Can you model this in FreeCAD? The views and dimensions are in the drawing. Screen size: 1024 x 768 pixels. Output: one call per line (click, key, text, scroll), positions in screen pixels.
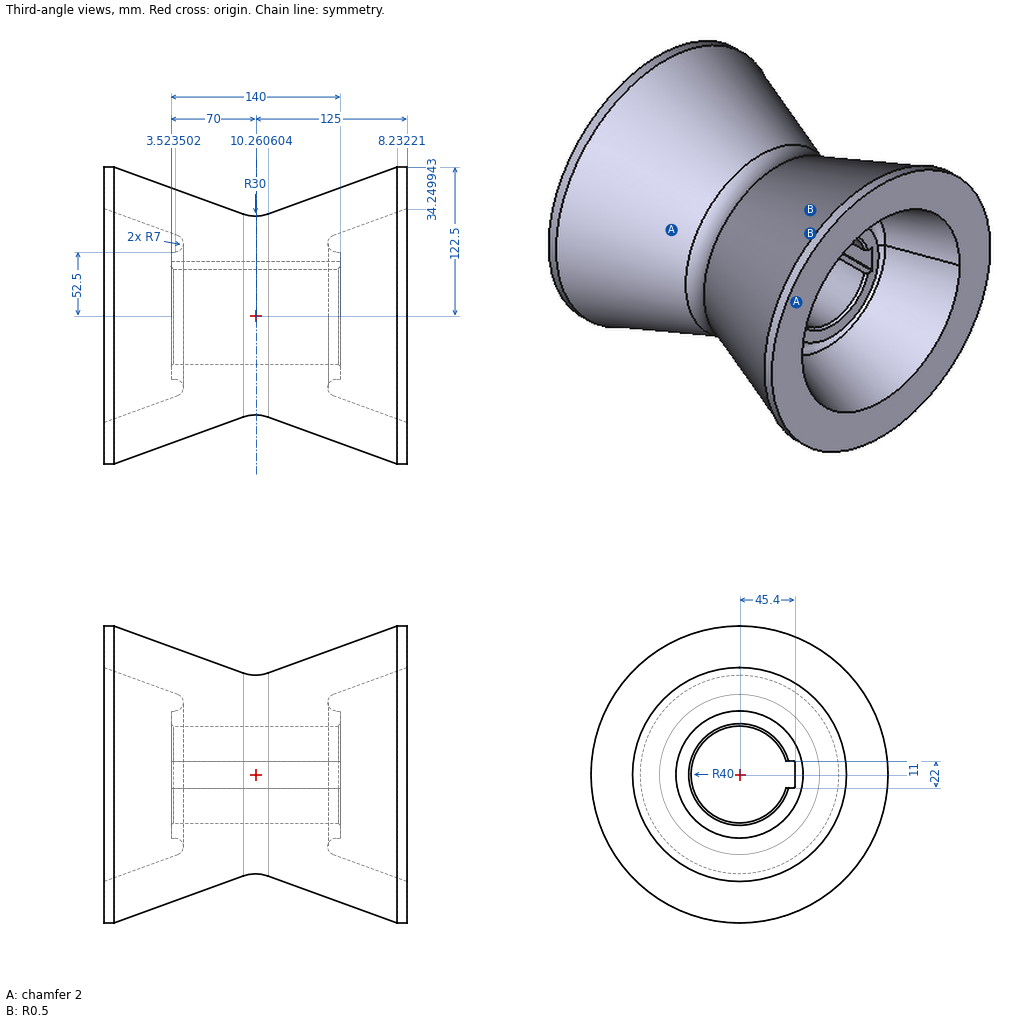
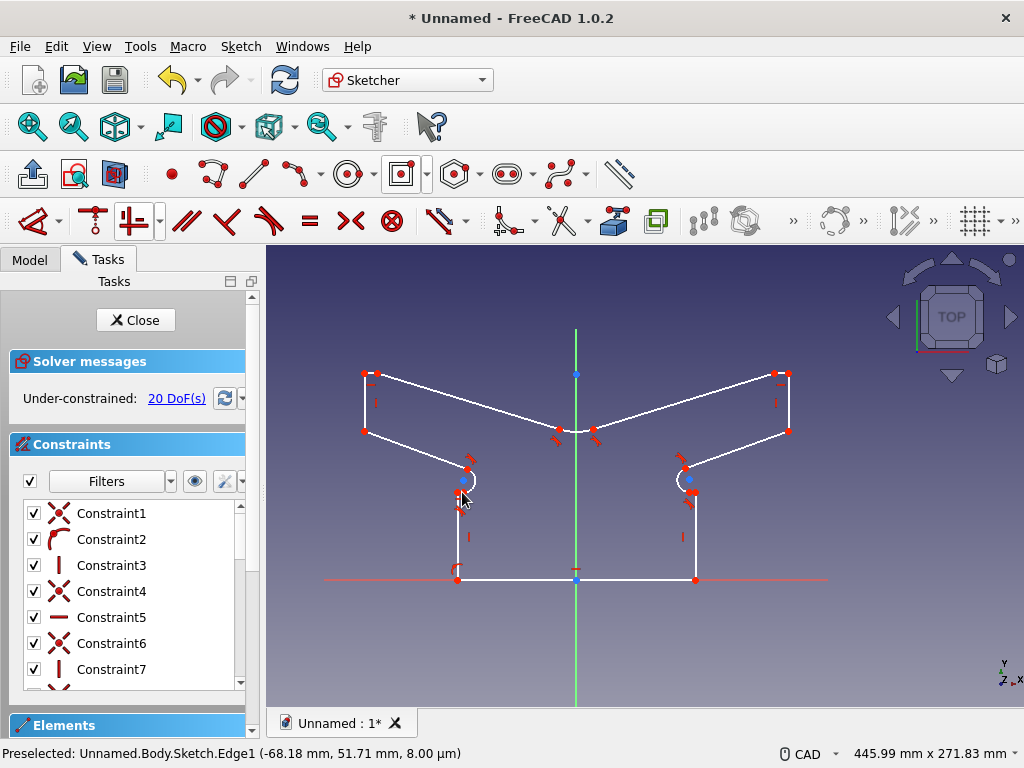
scroll(693, 492, up, 9)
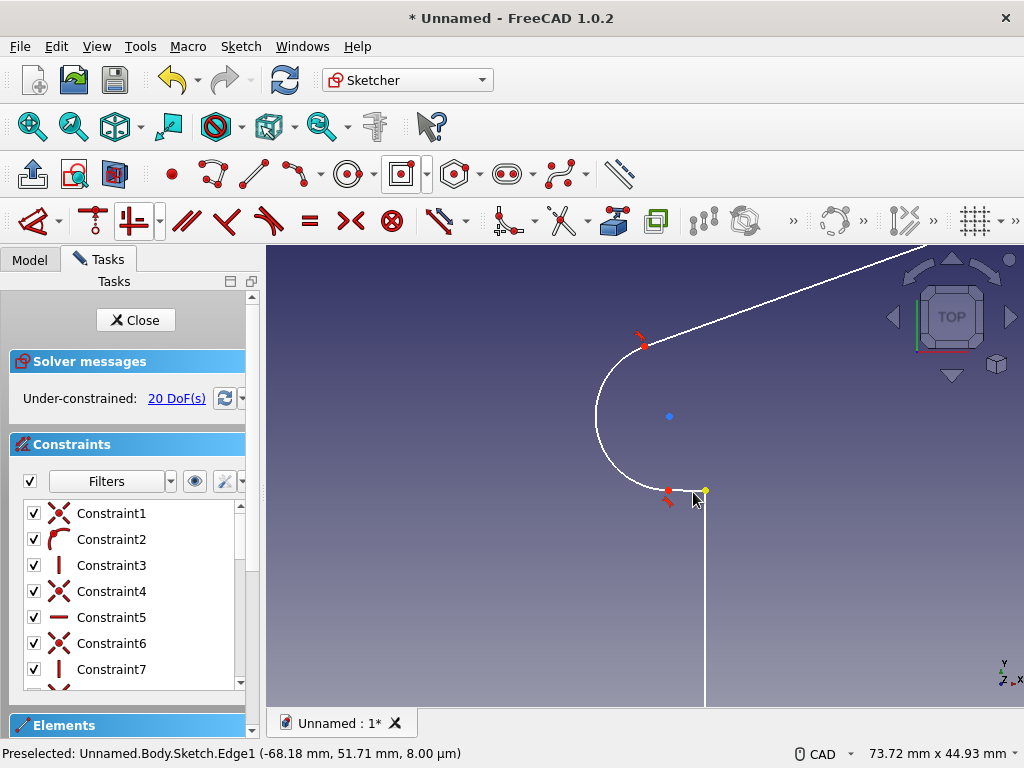
click(691, 491)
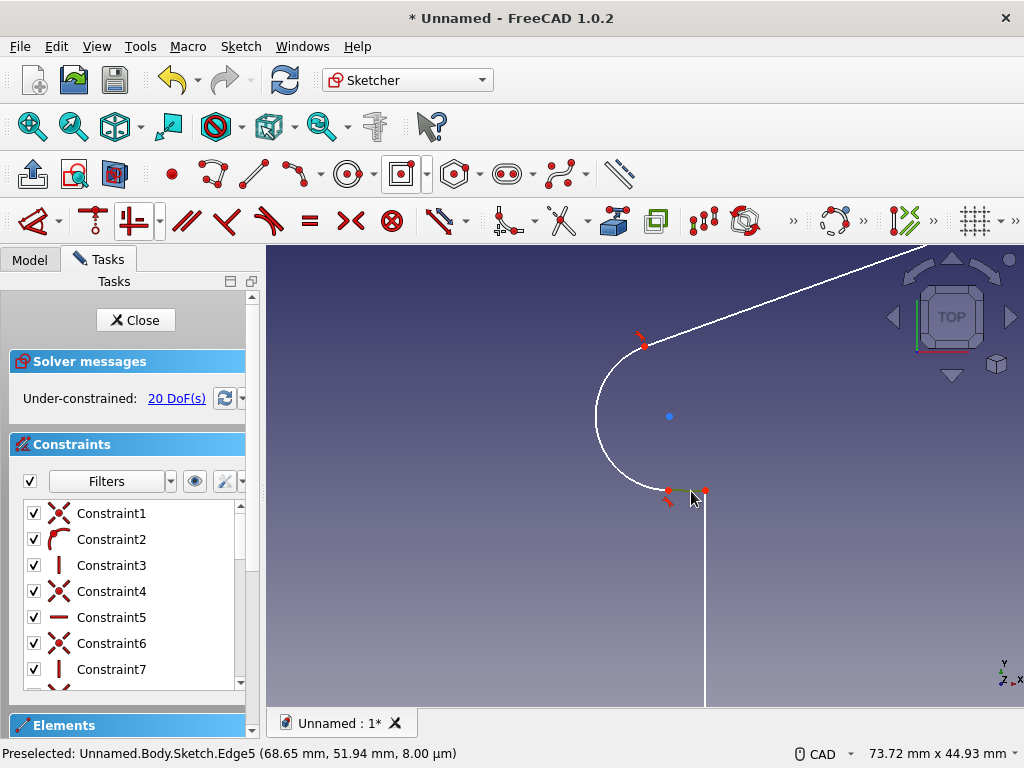
key(h)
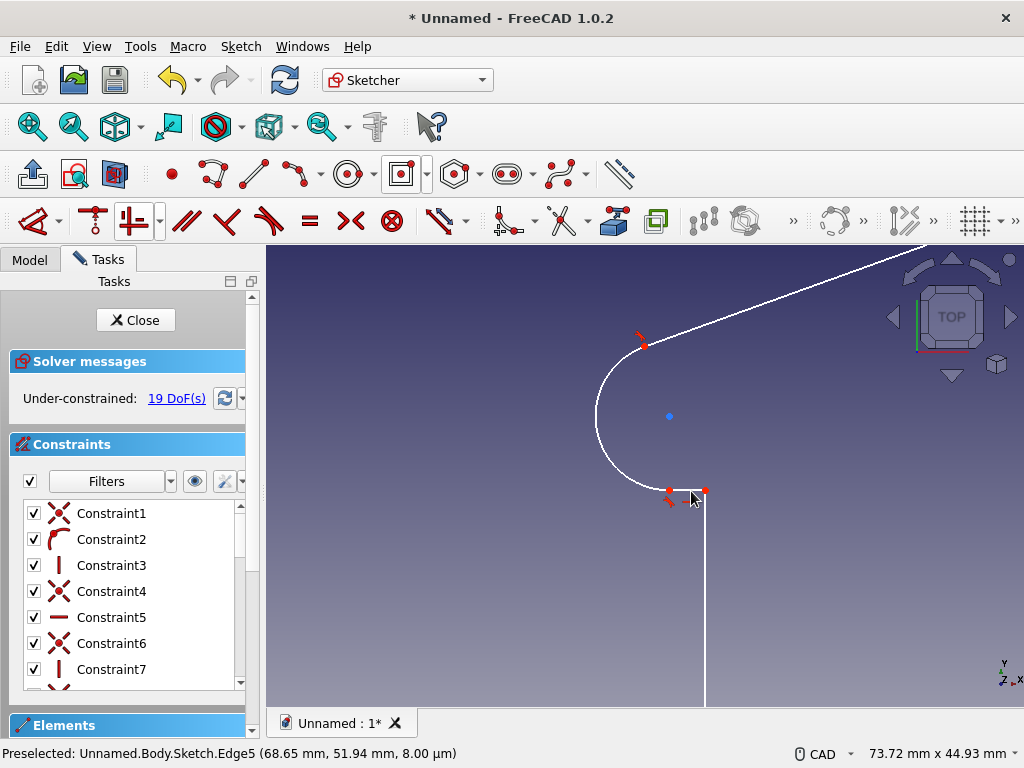
scroll(694, 492, down, 9)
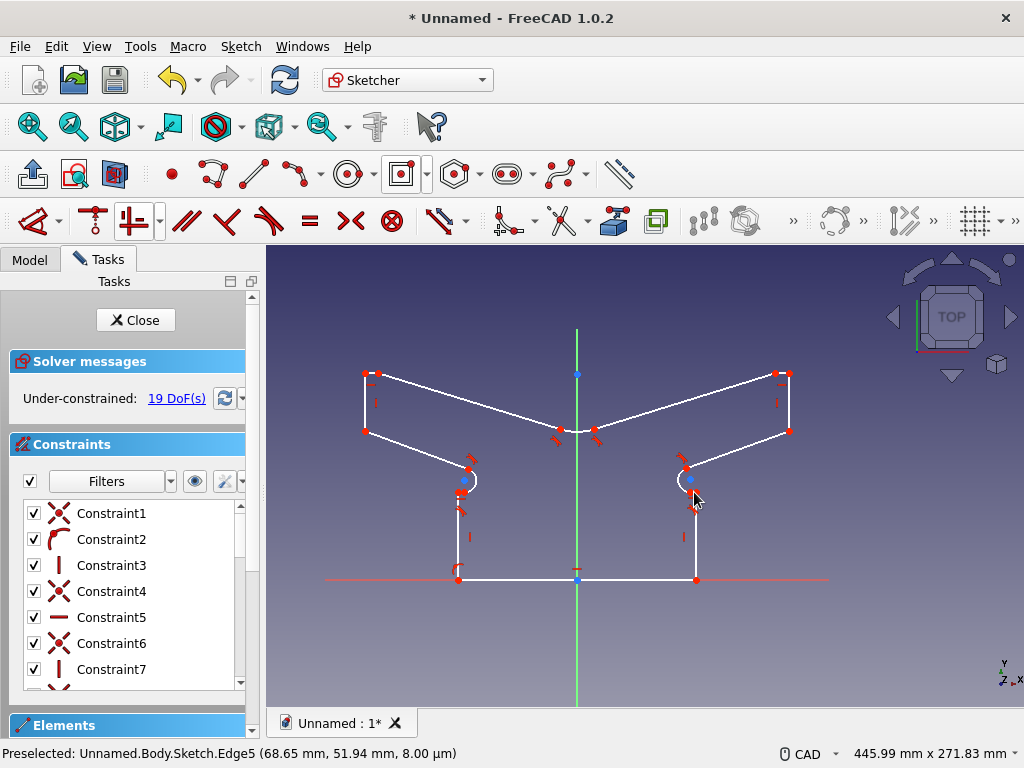
scroll(679, 475, up, 2)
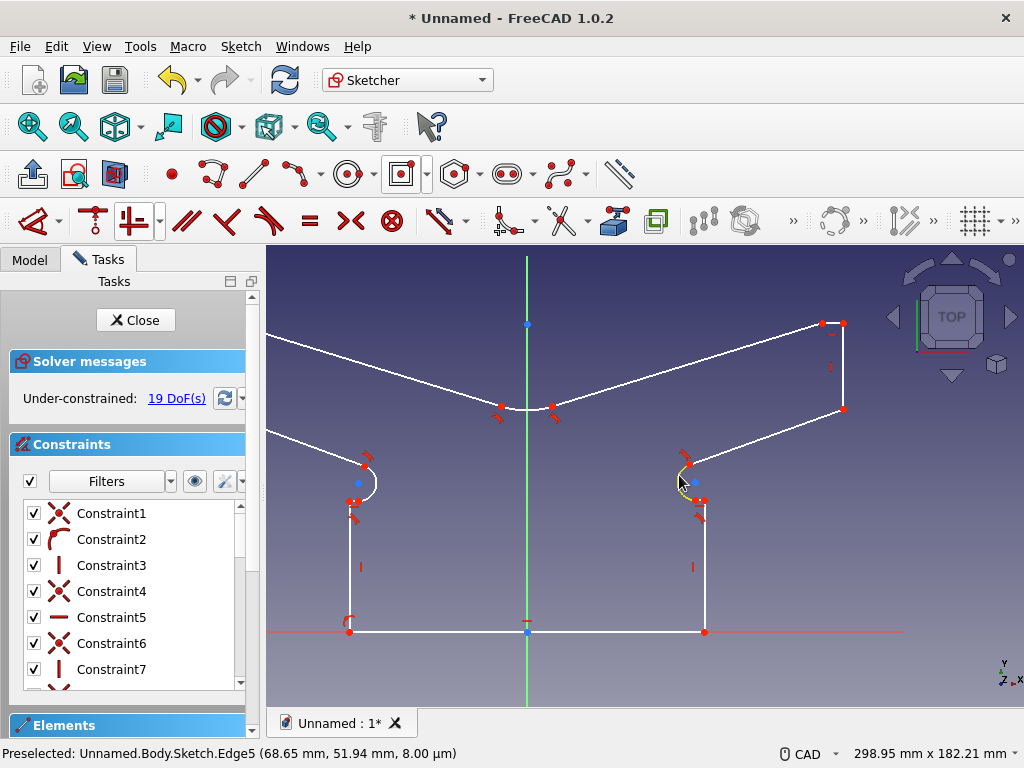
click(679, 475)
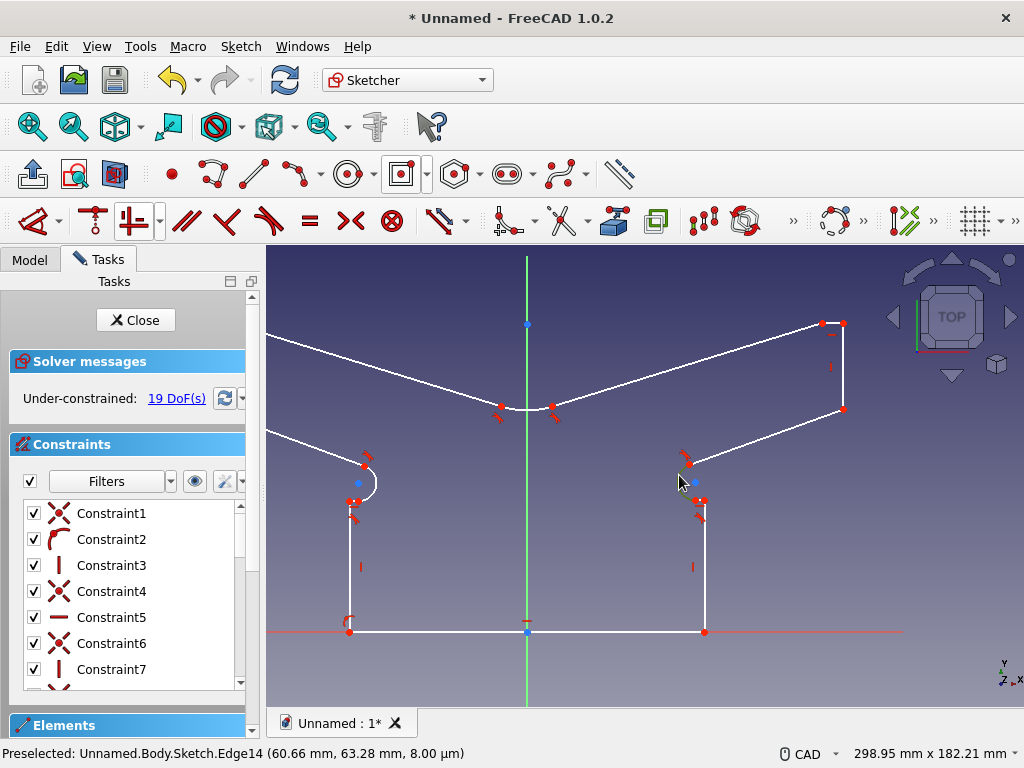
click(372, 495)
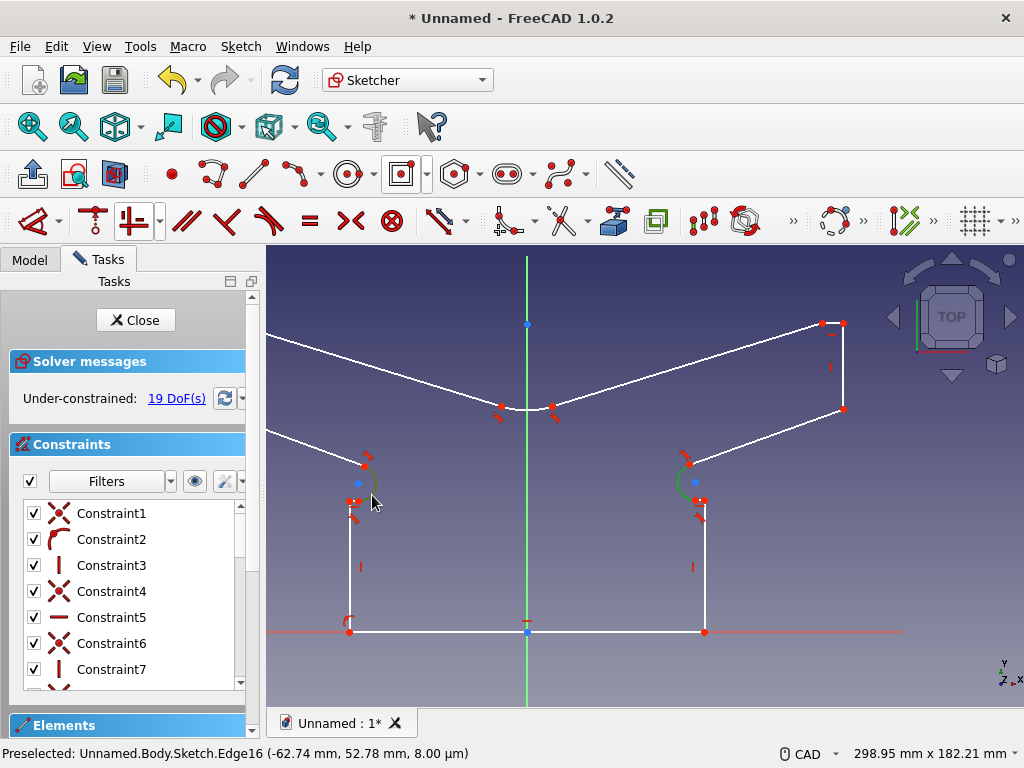
click(310, 222)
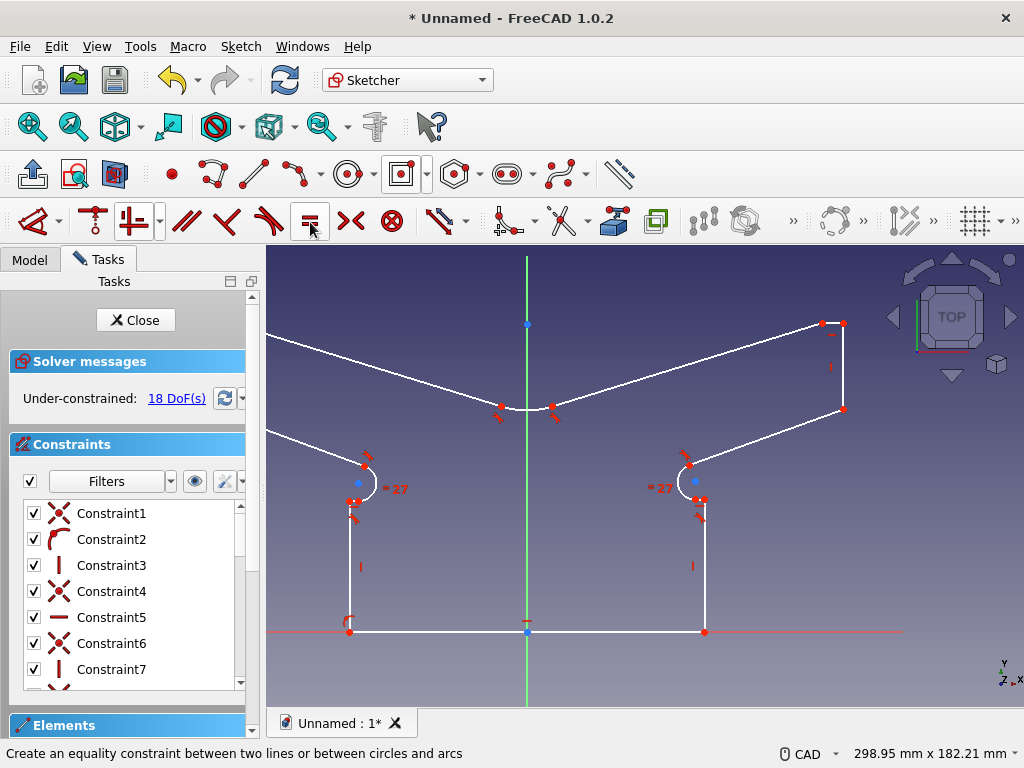
click(527, 324)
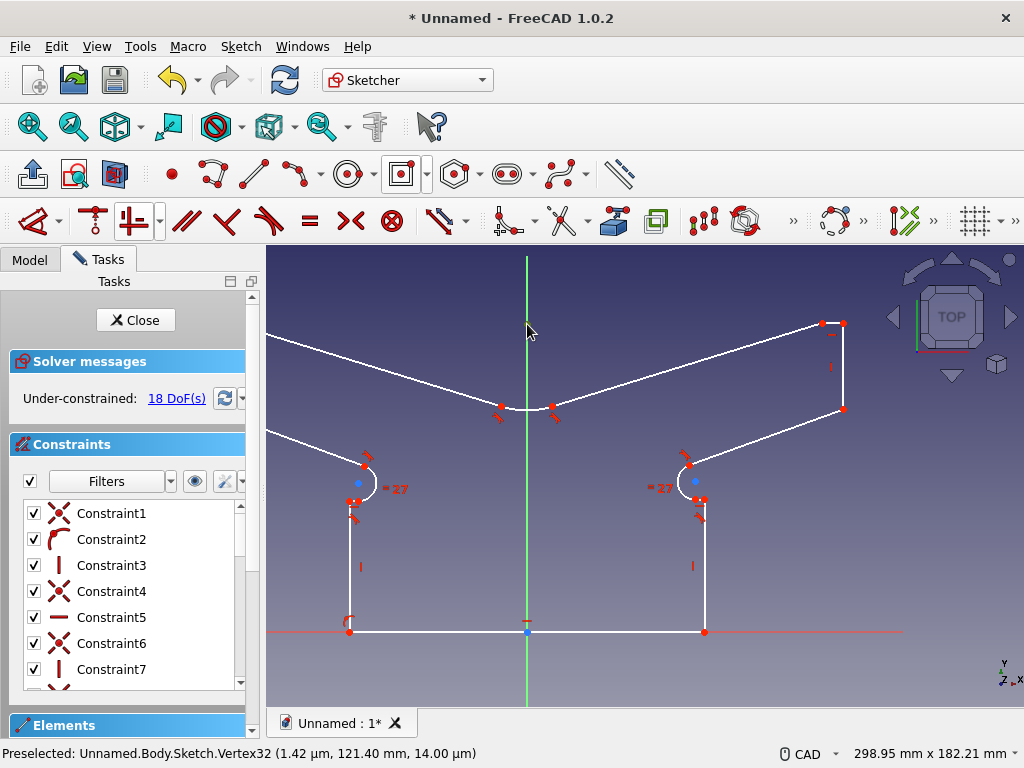
click(527, 592)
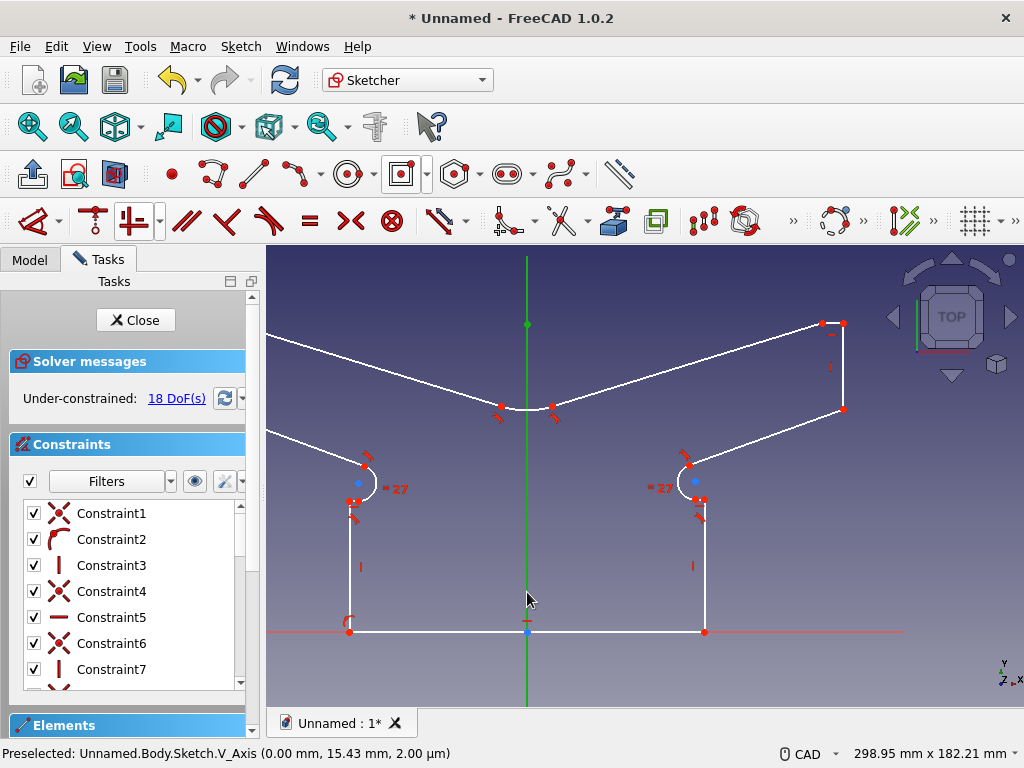
click(93, 222)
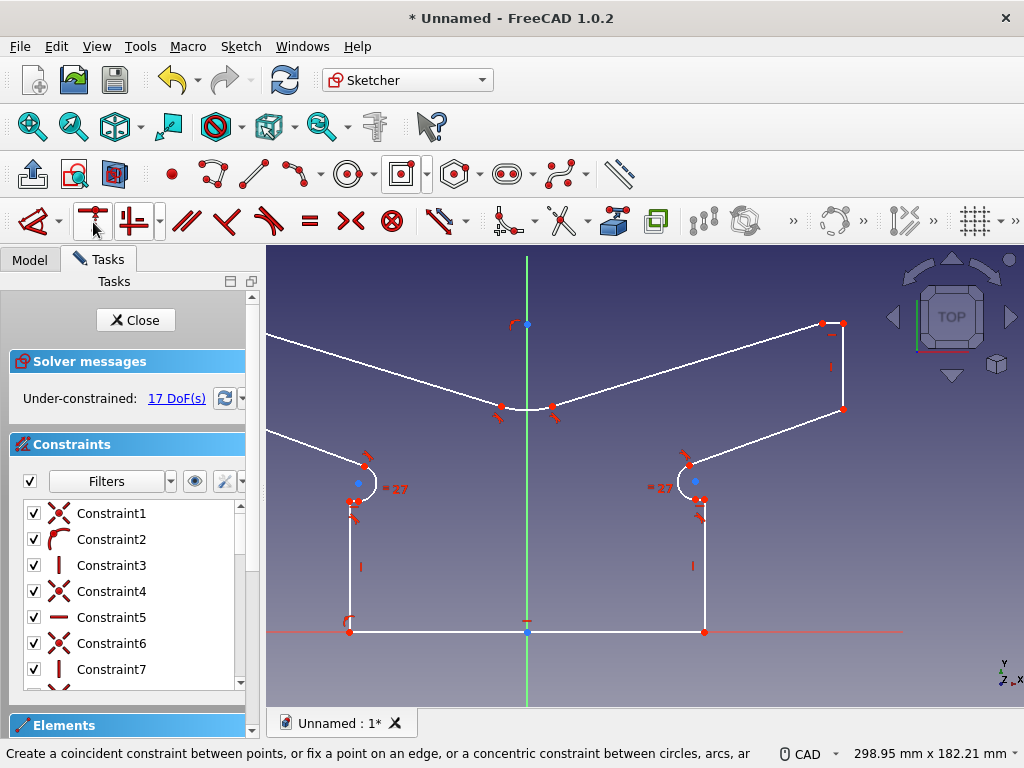
click(696, 482)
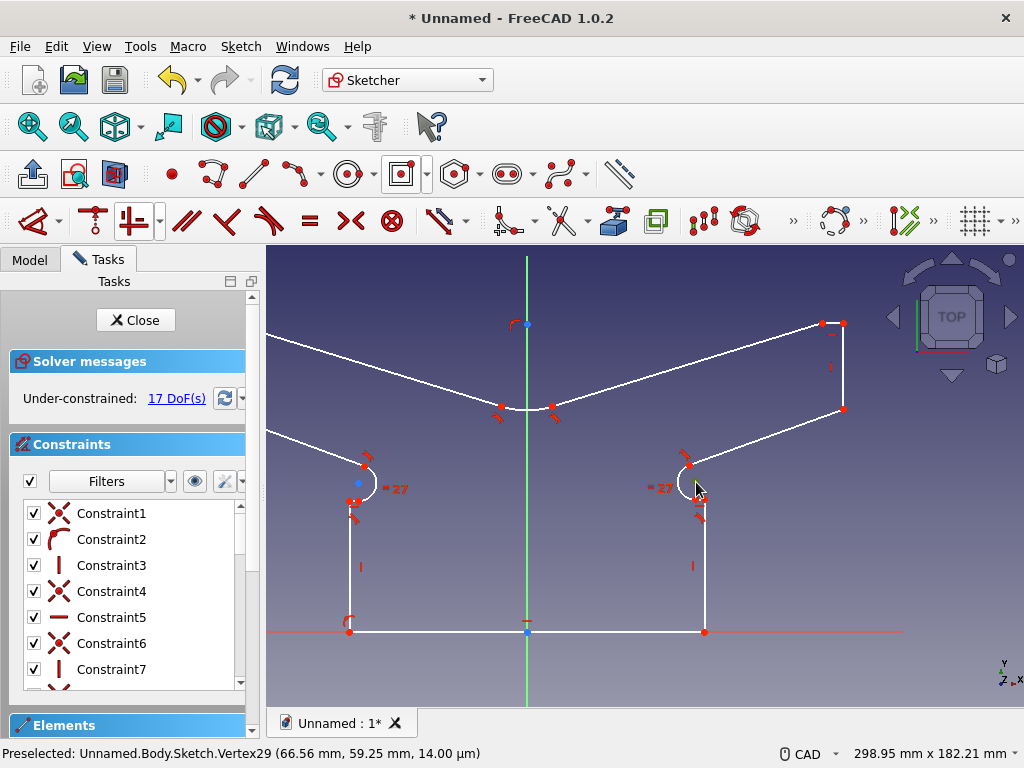
click(358, 483)